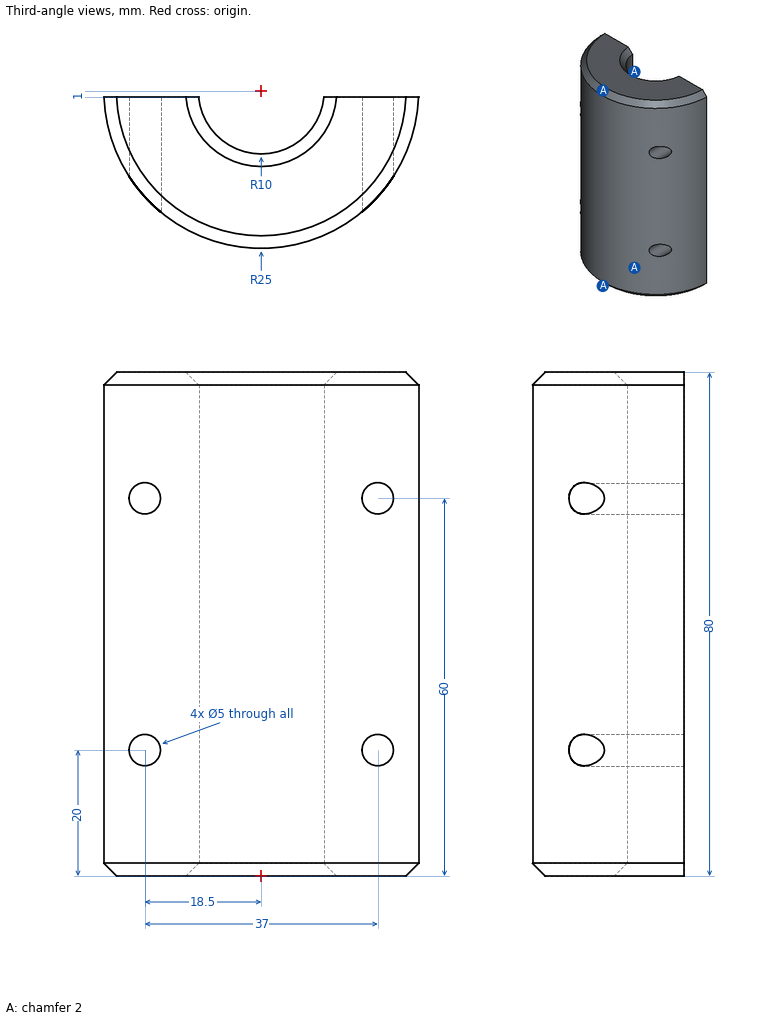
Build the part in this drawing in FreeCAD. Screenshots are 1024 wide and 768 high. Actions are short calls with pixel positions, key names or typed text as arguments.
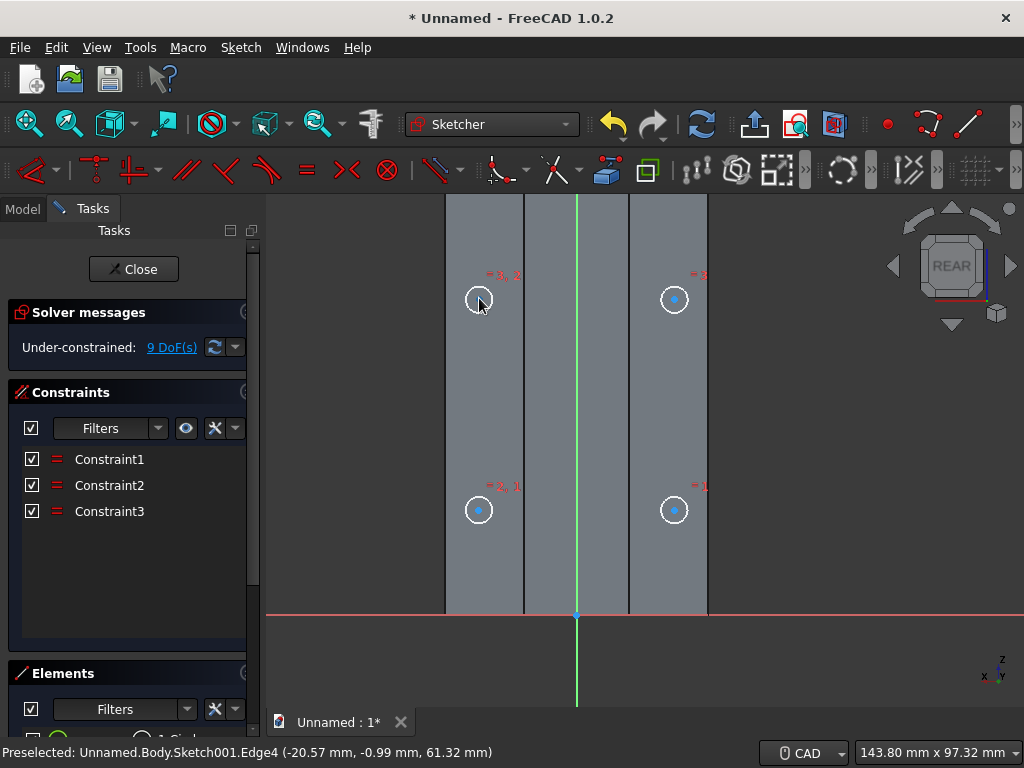
click(674, 510)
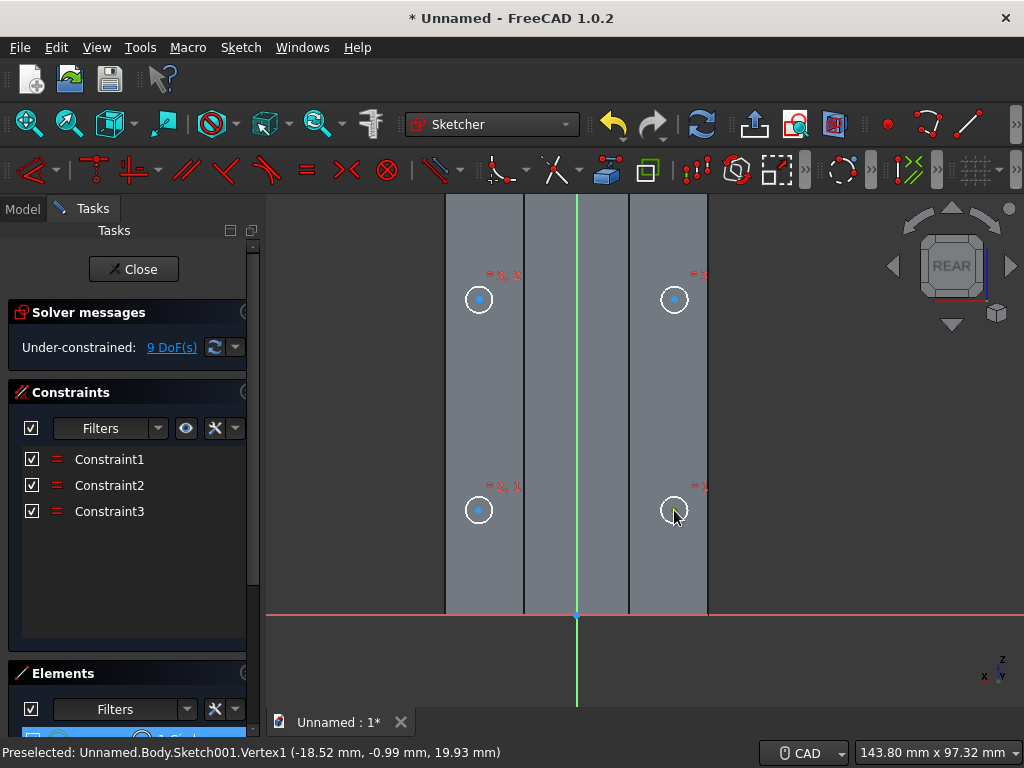
click(479, 510)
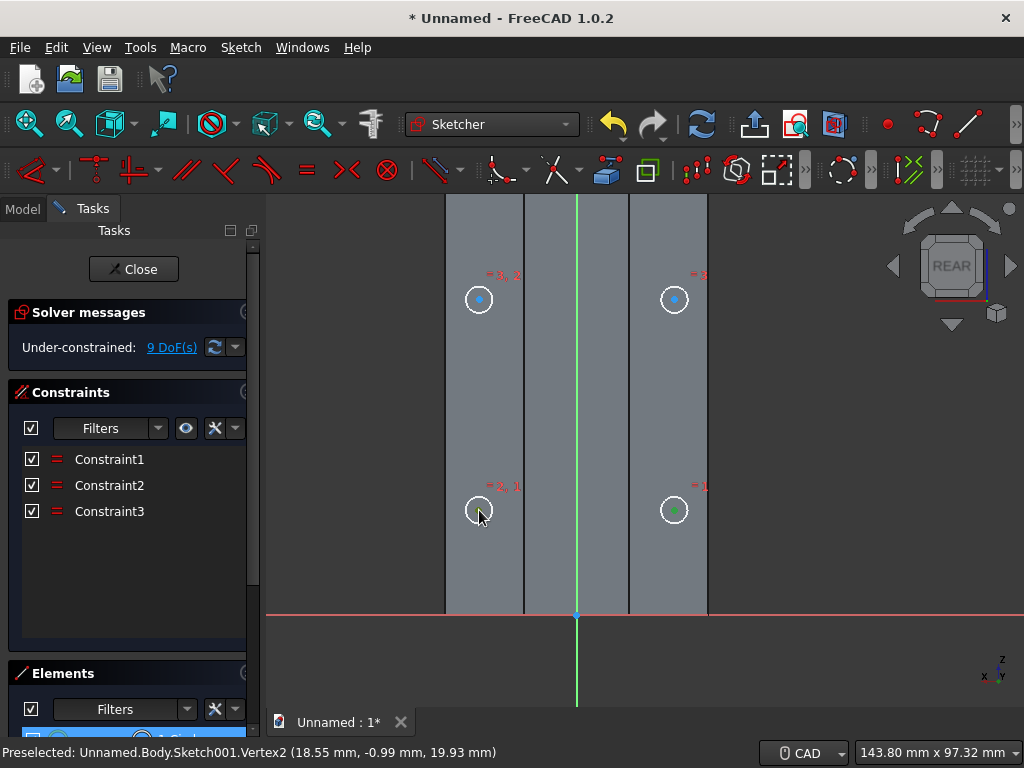
click(160, 170)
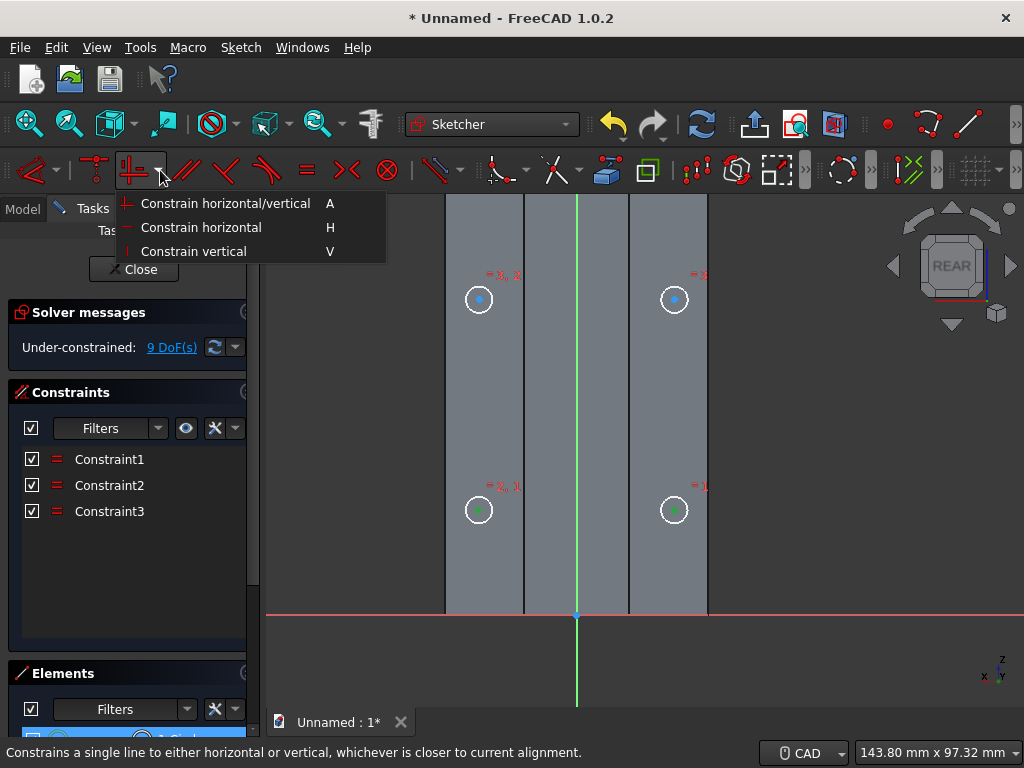
click(251, 227)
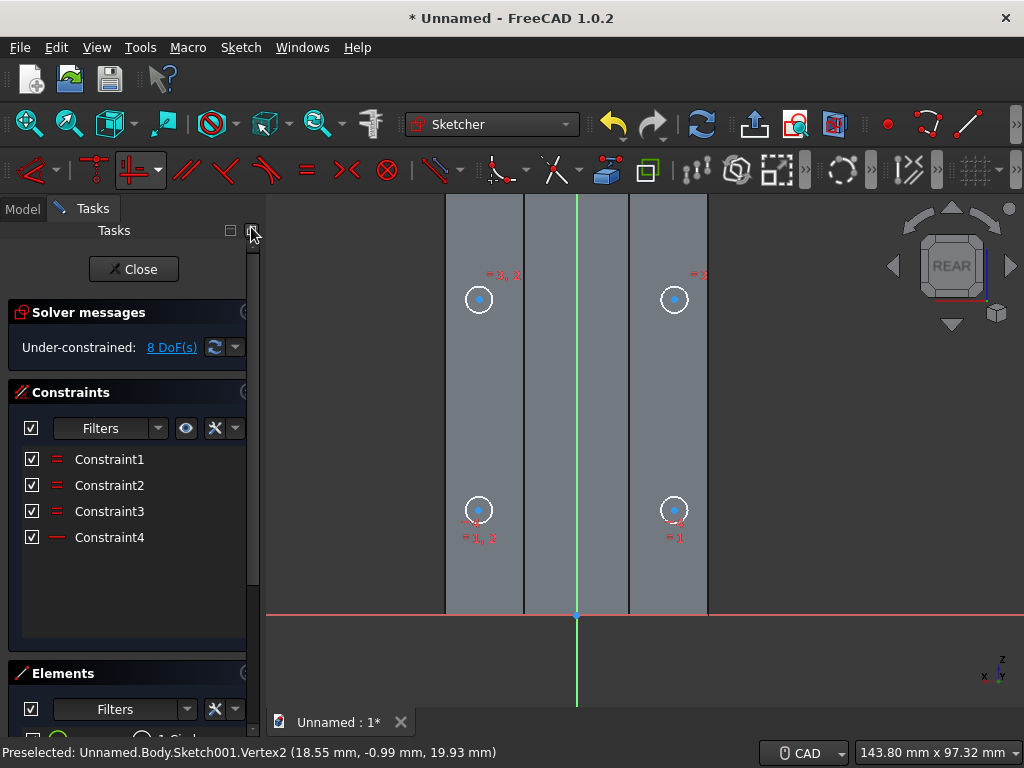
click(479, 510)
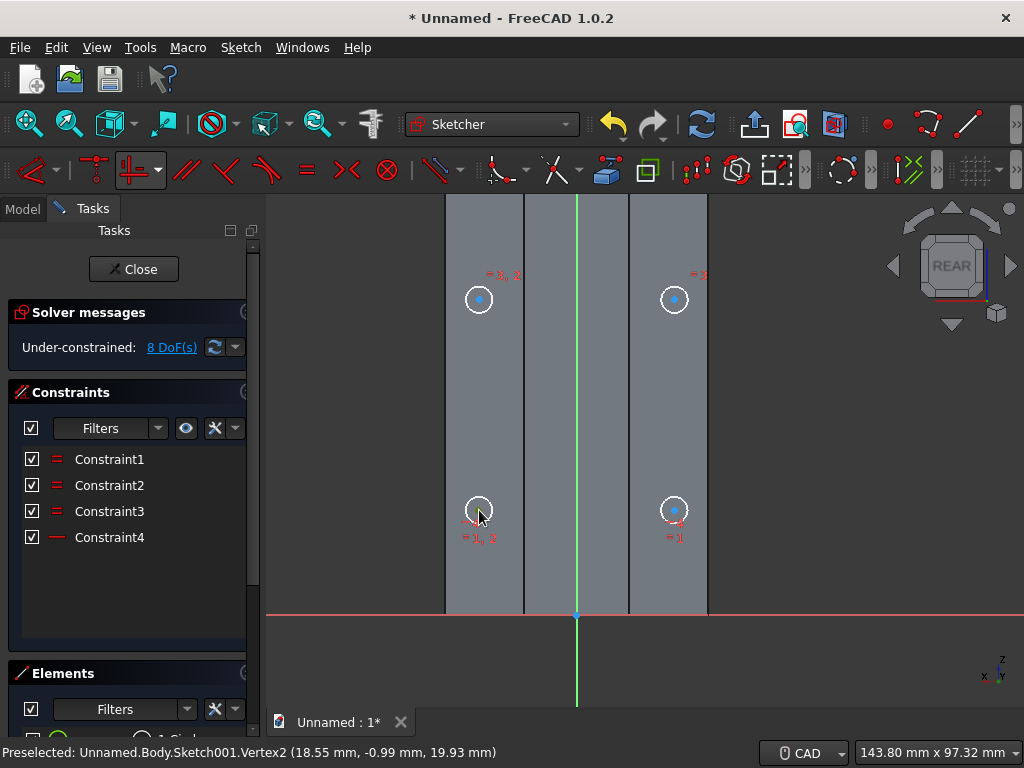
click(479, 300)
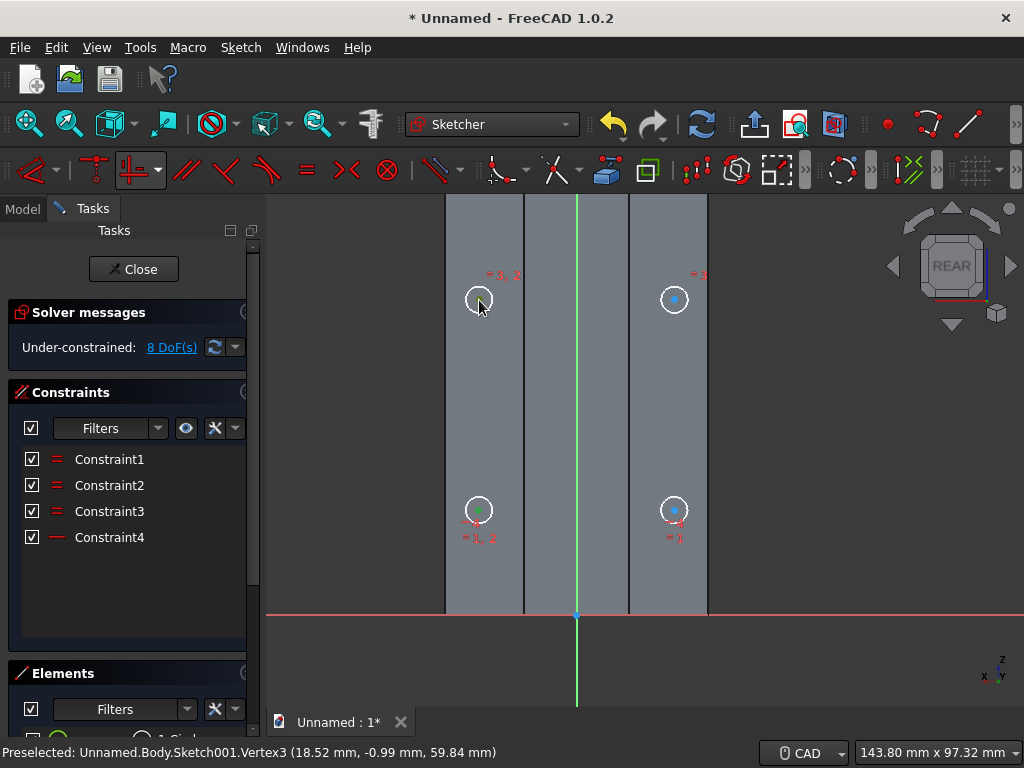
key(v)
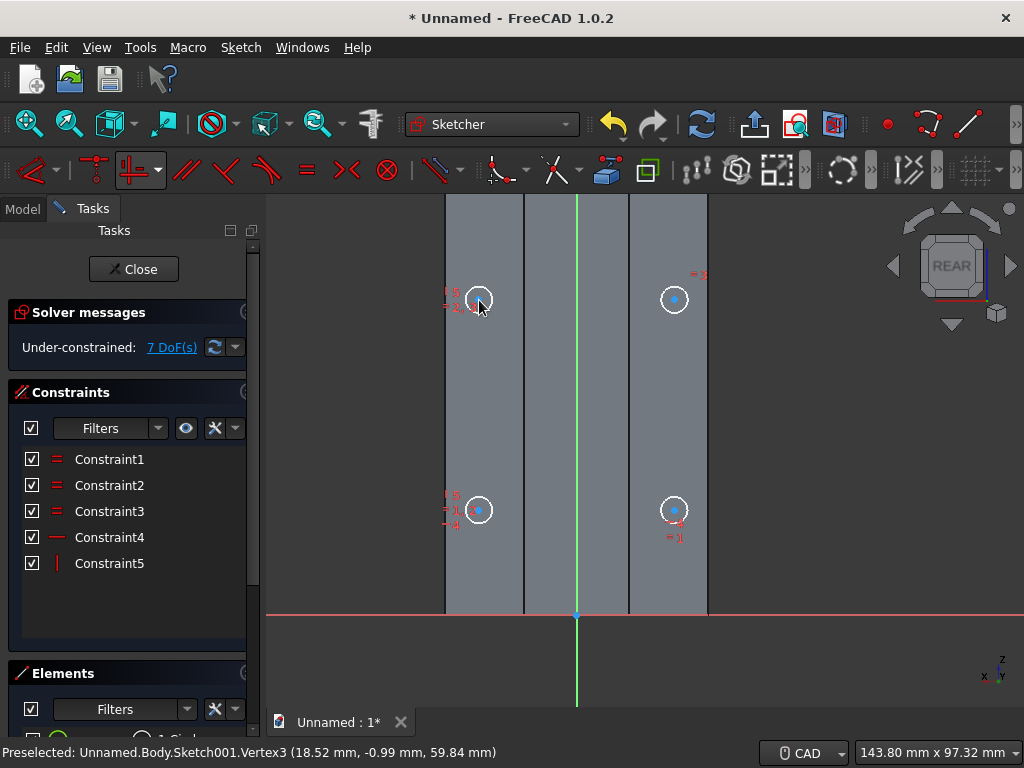
click(674, 510)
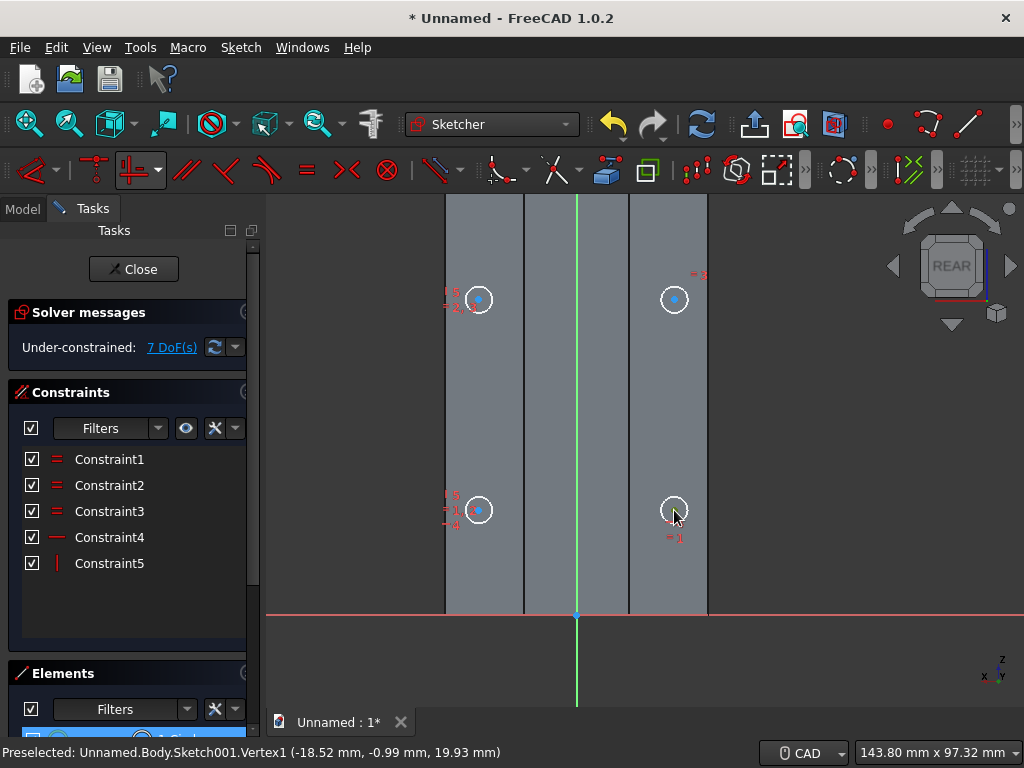
click(675, 300)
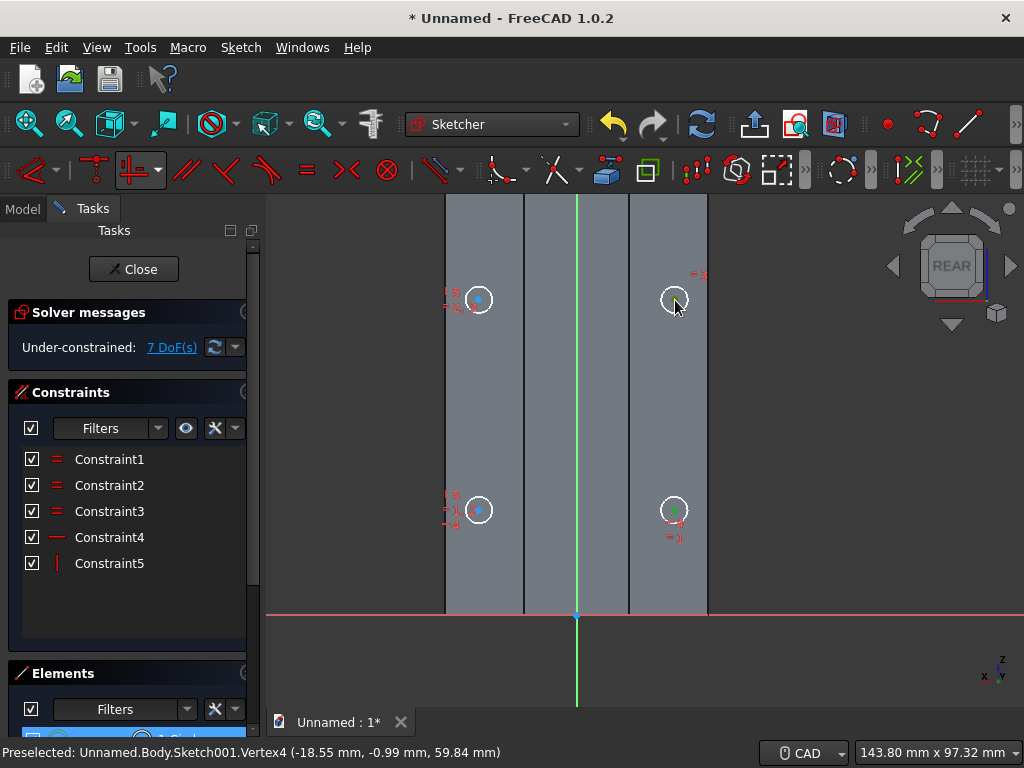
click(160, 170)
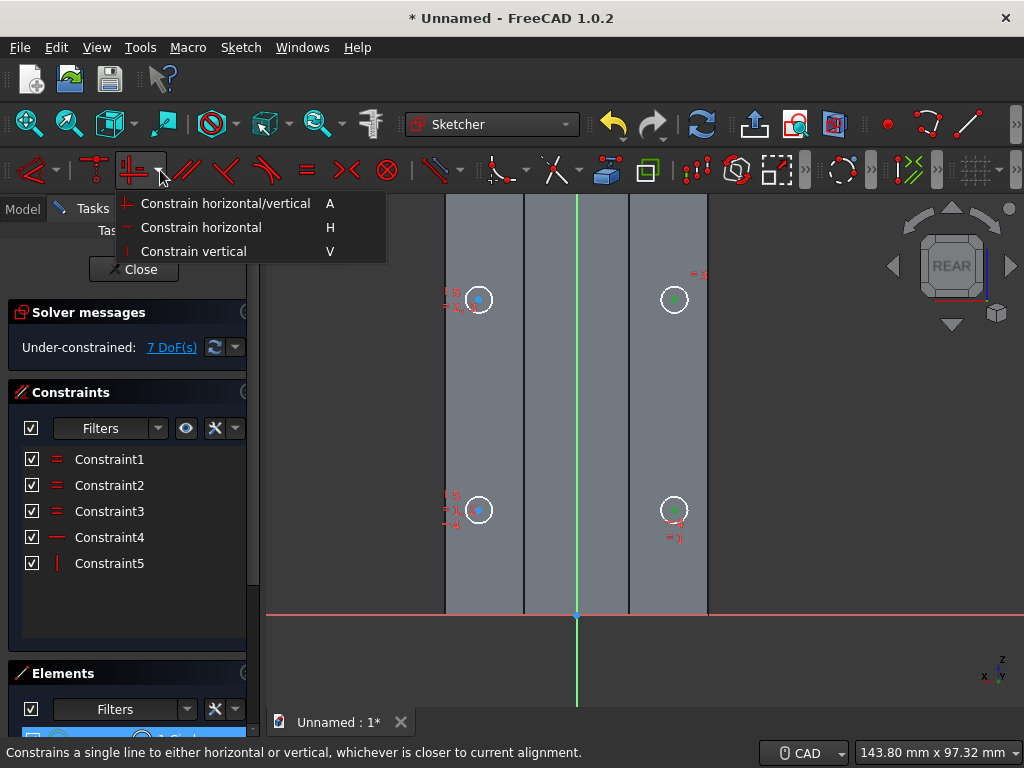
click(251, 251)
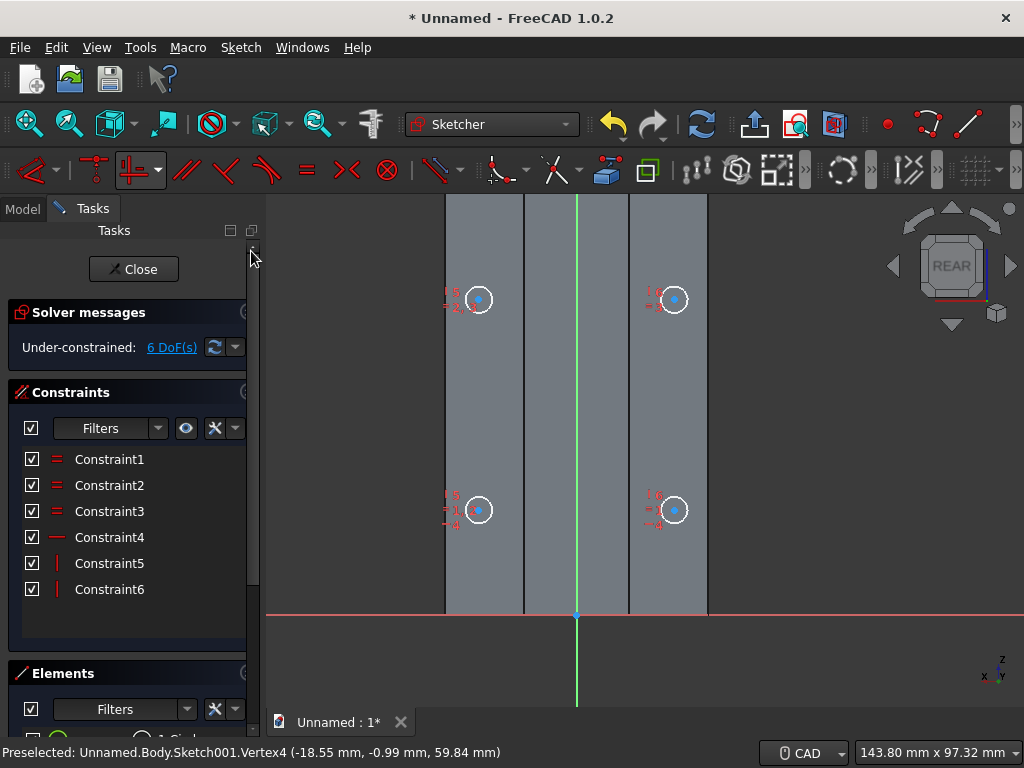
click(479, 300)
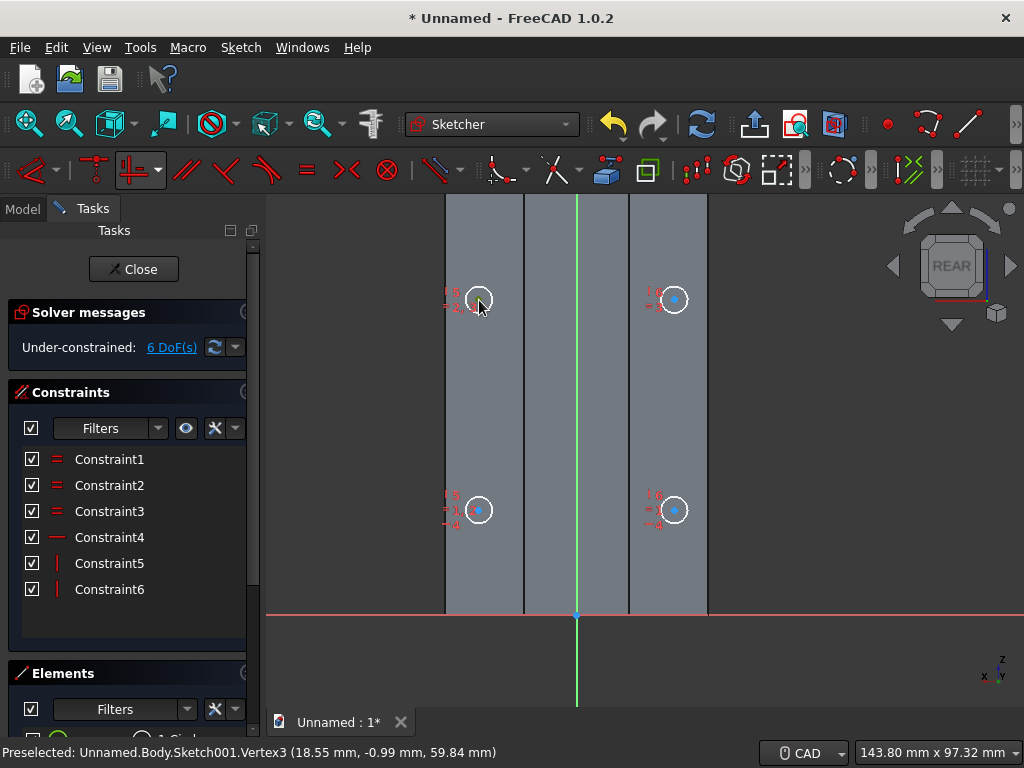
click(674, 300)